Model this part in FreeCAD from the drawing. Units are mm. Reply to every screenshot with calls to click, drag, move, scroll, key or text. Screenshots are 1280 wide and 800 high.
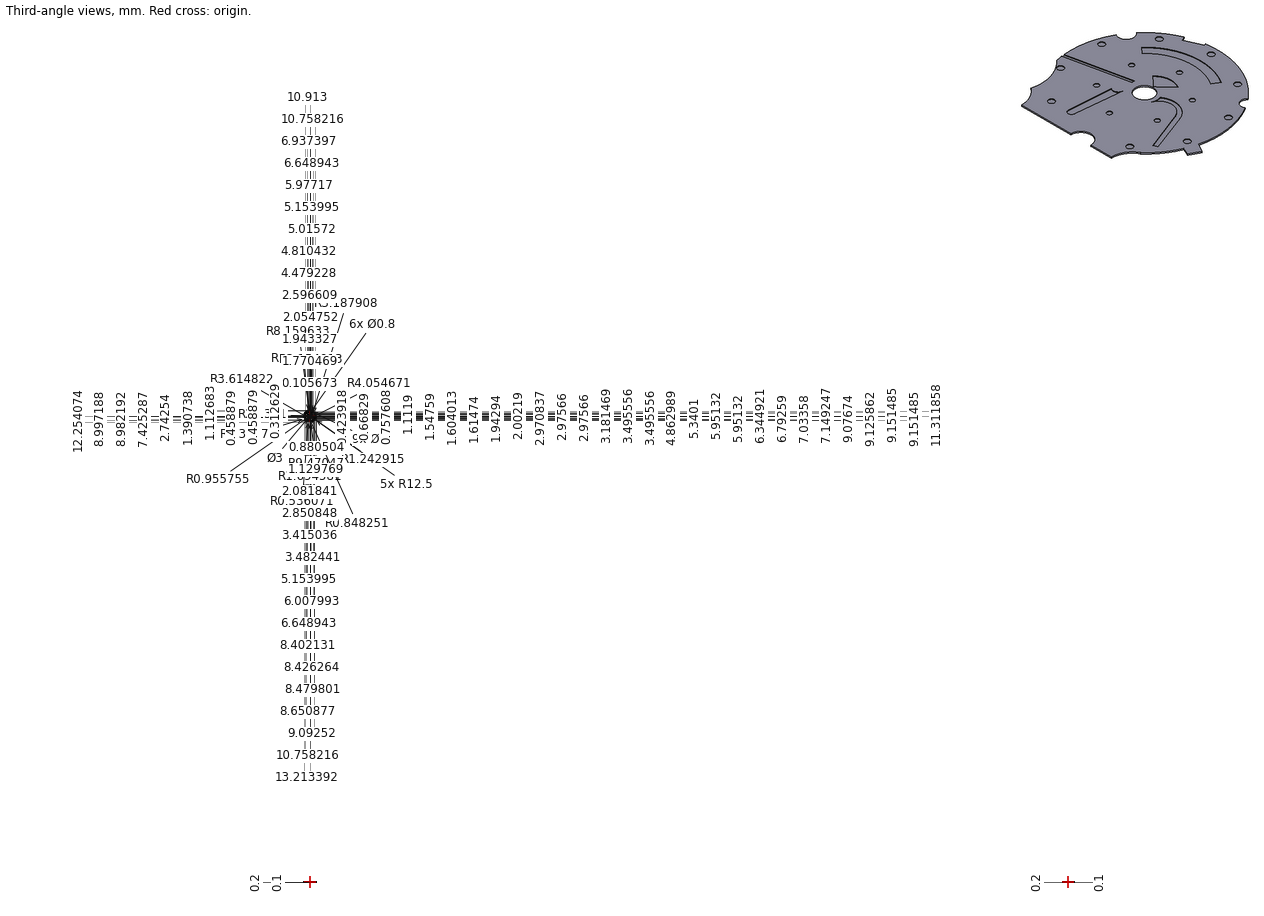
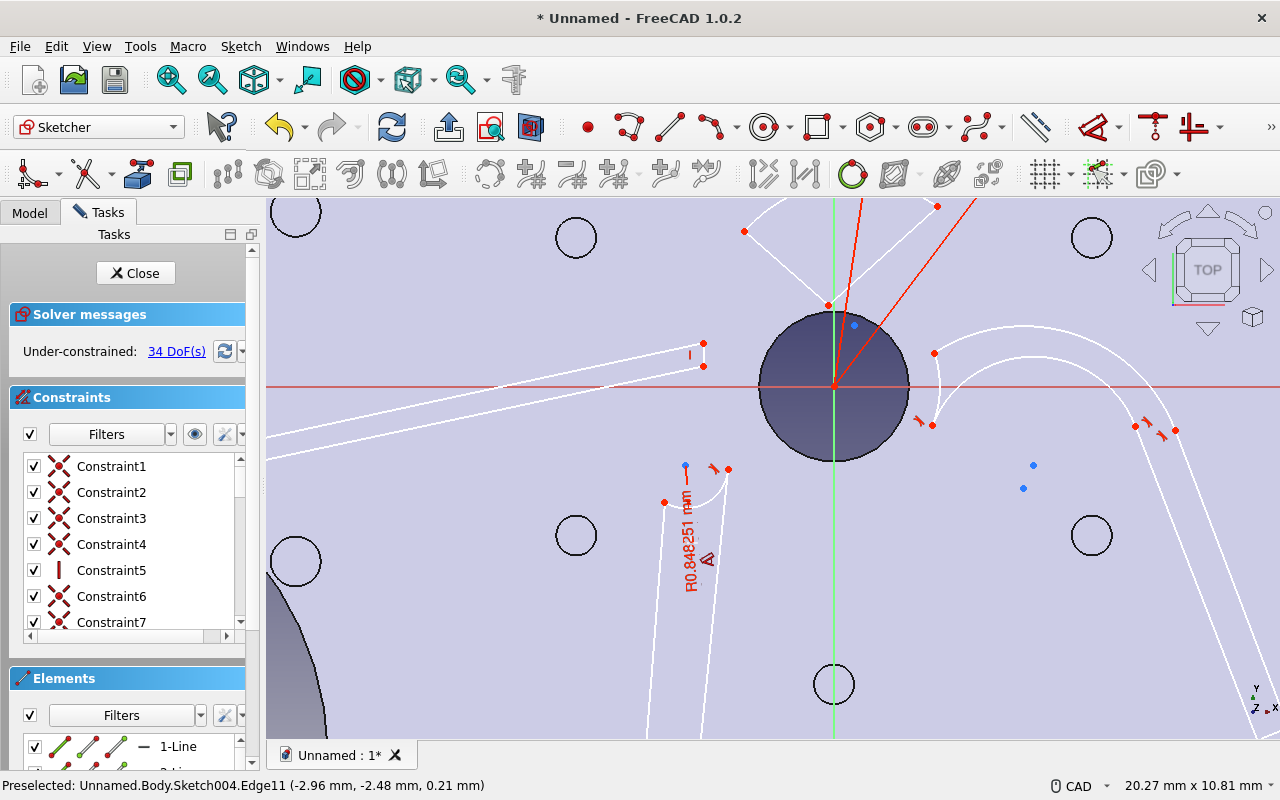
scroll(689, 513, down, 5)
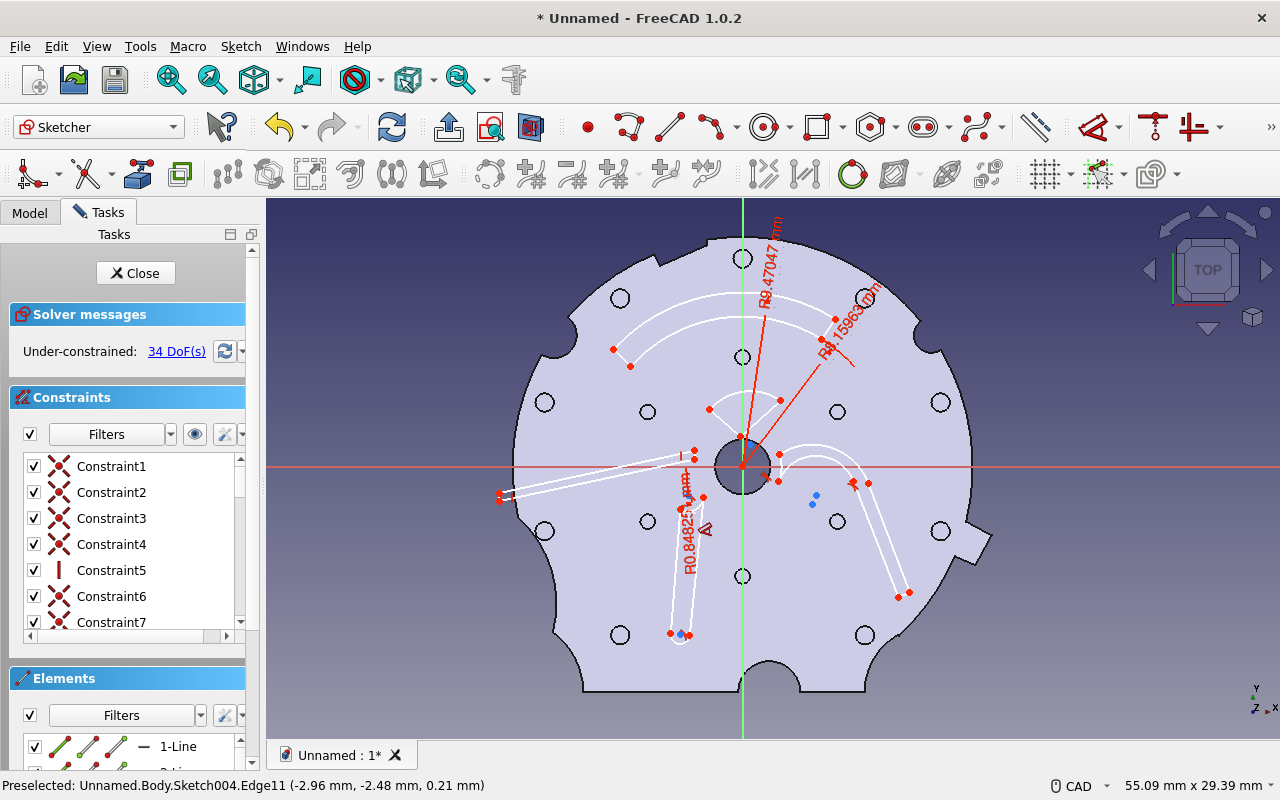
scroll(674, 642, up, 7)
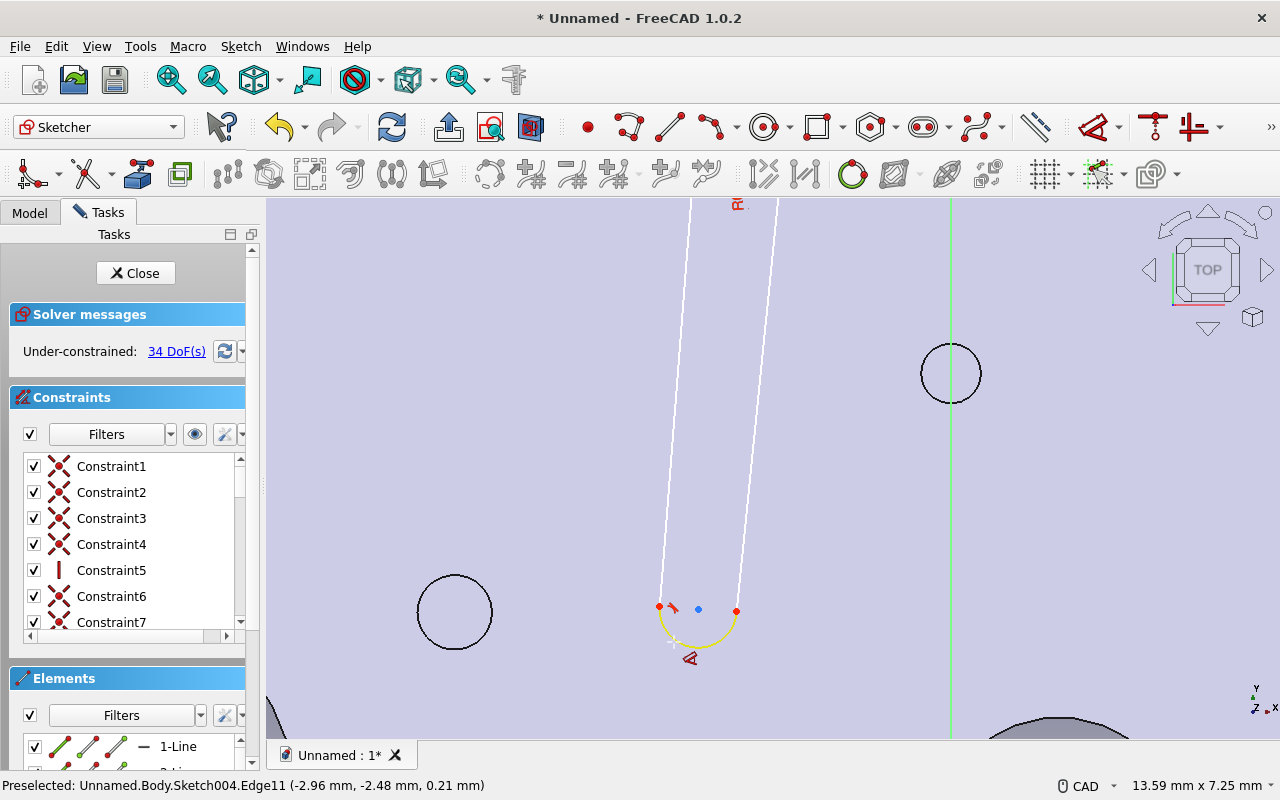
click(673, 639)
click(652, 663)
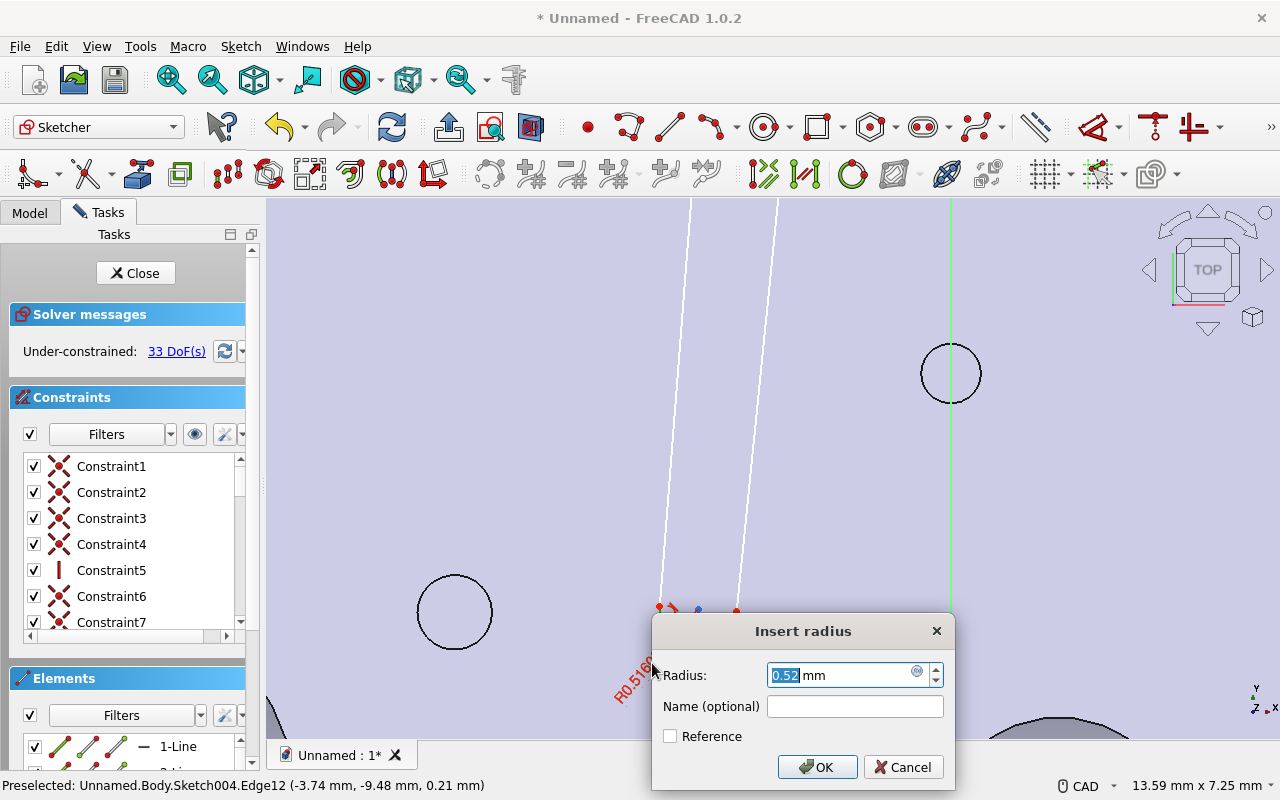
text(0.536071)
key(Return)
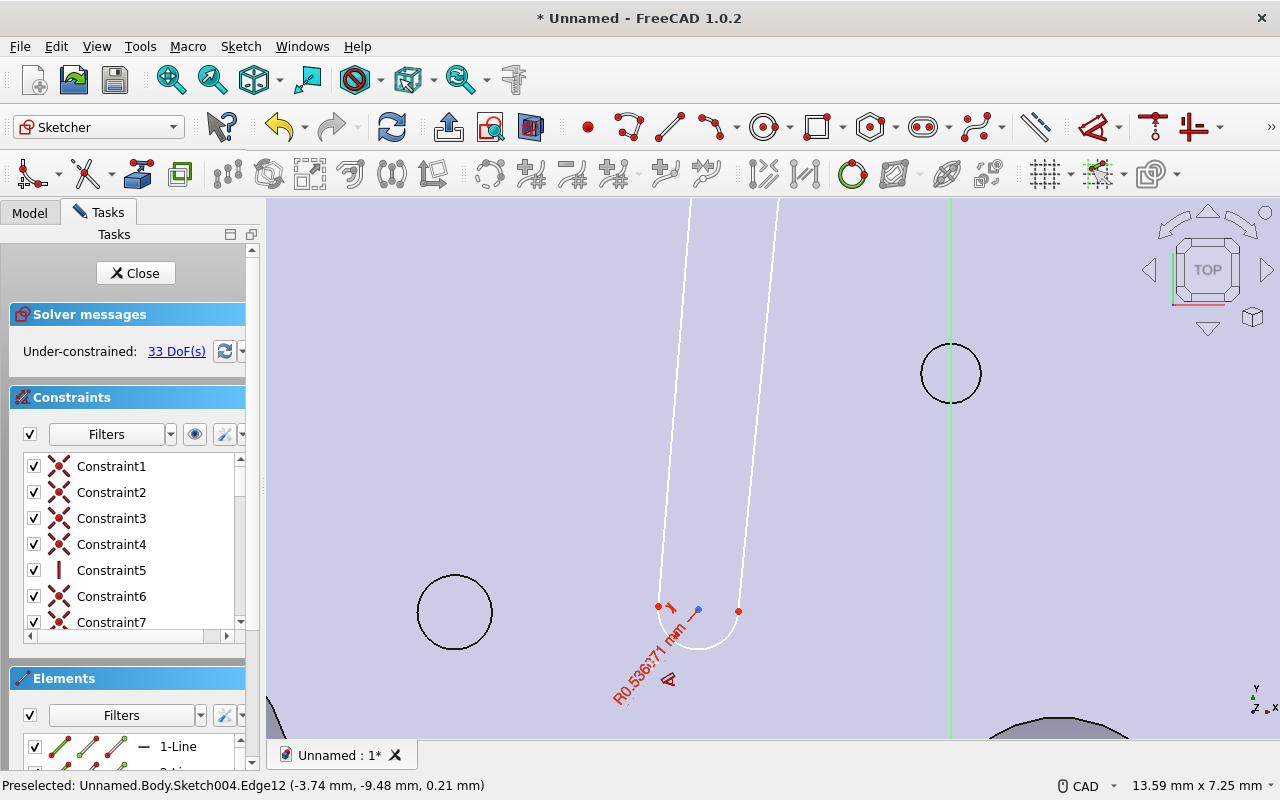
scroll(674, 643, down, 7)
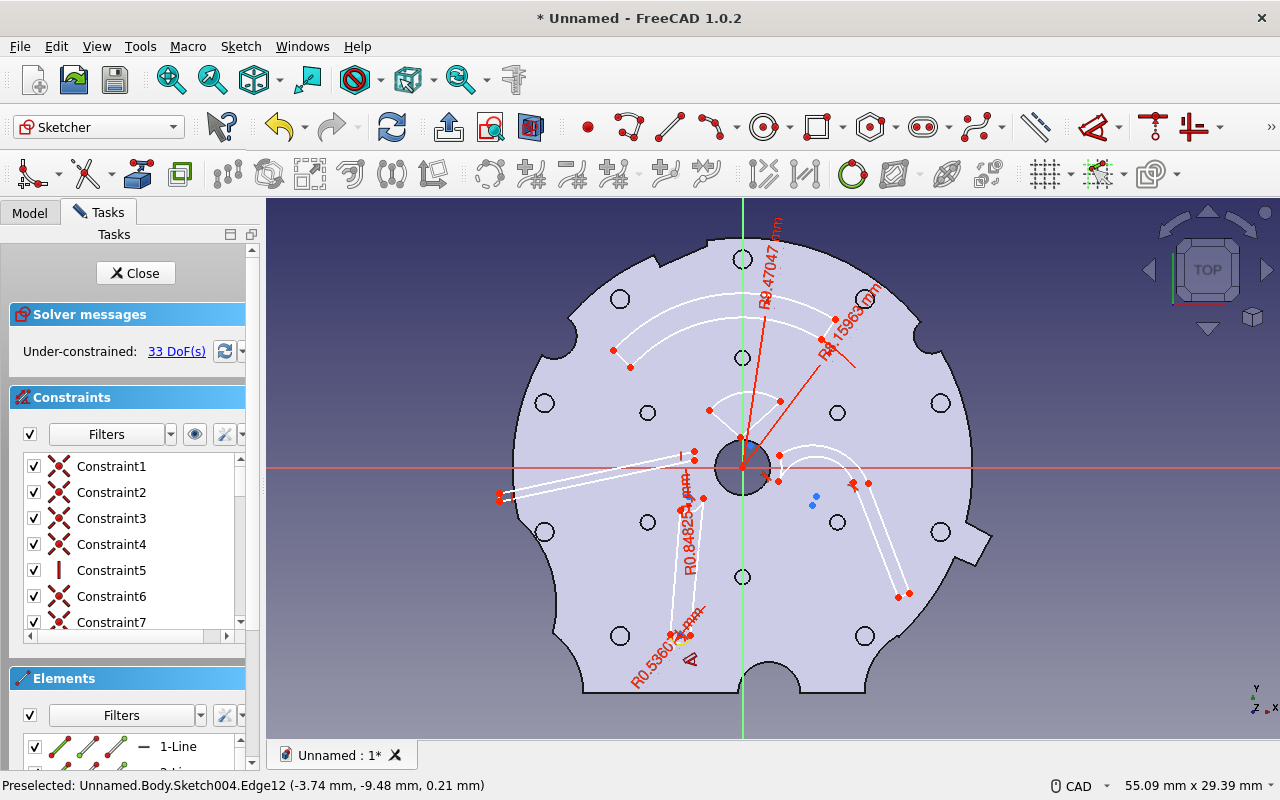
click(759, 393)
click(764, 361)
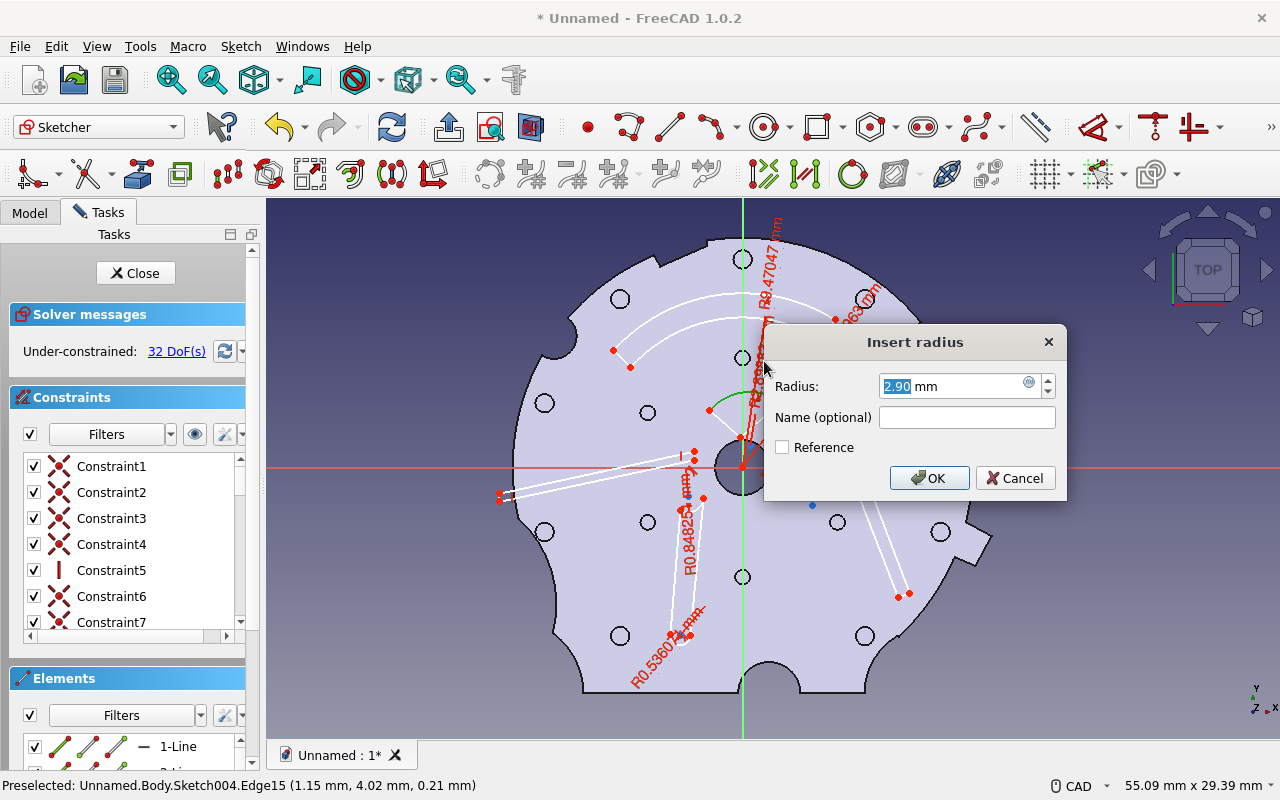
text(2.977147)
key(Return)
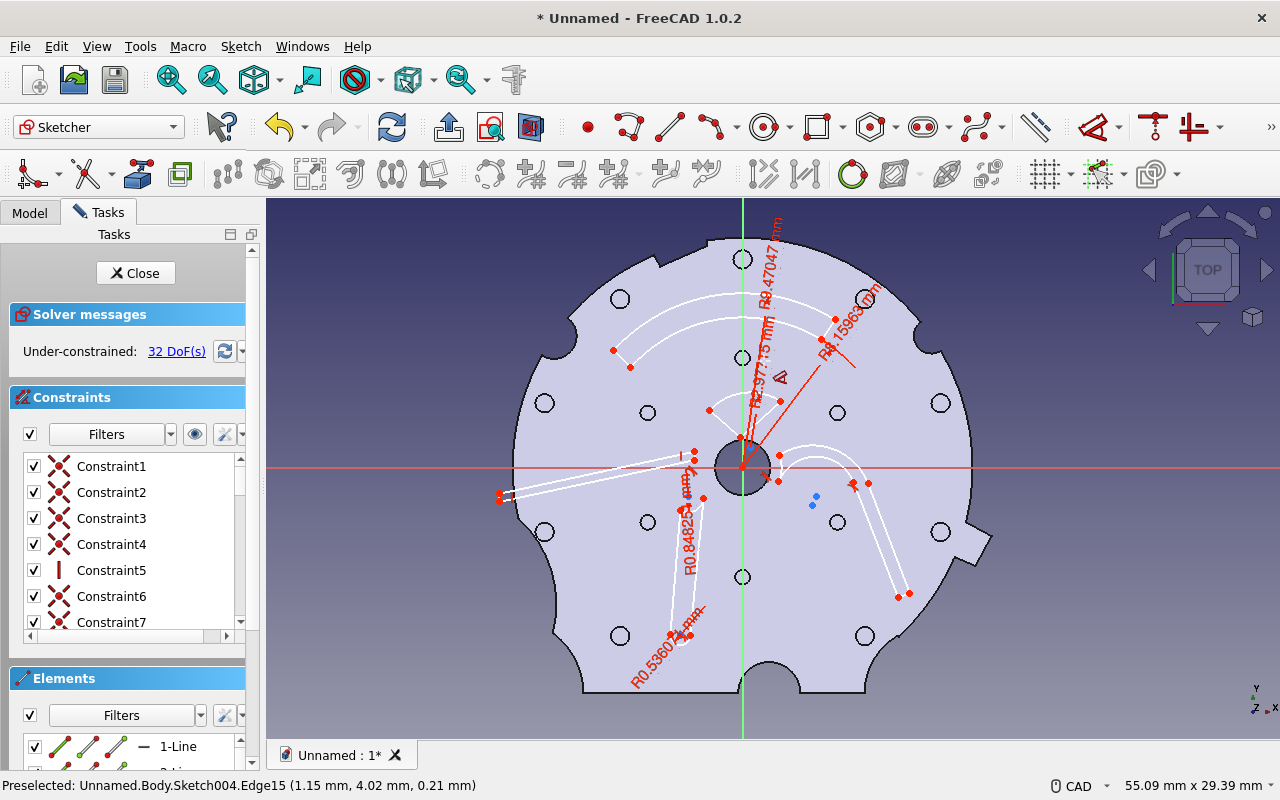
scroll(849, 458, up, 2)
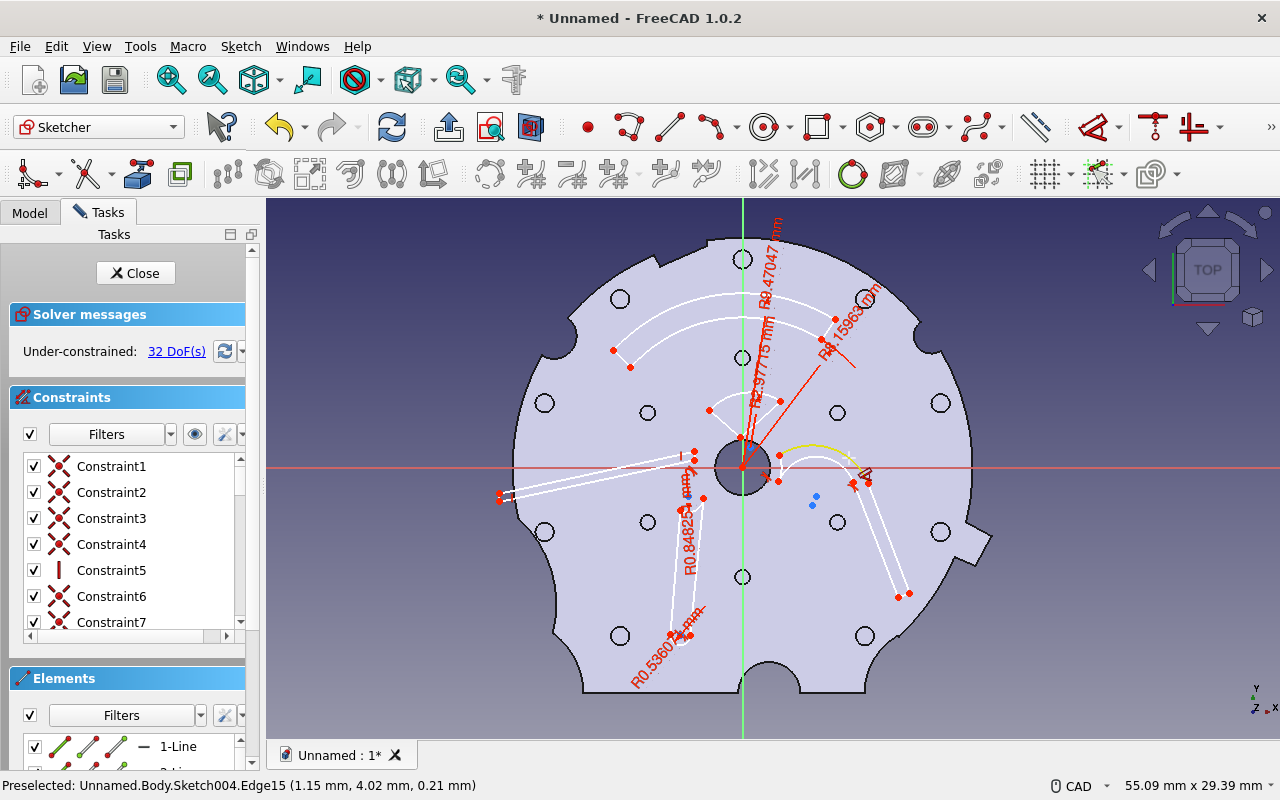
click(849, 458)
click(869, 433)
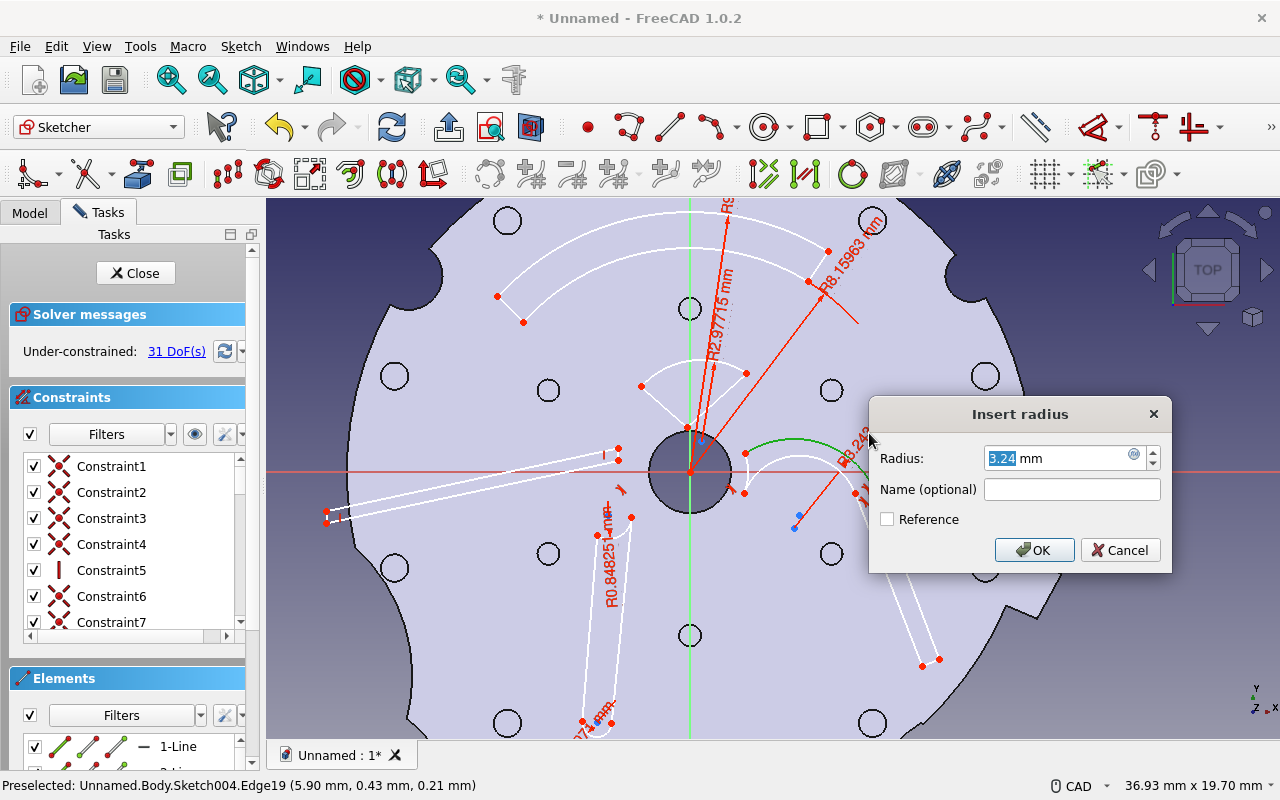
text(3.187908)
key(Return)